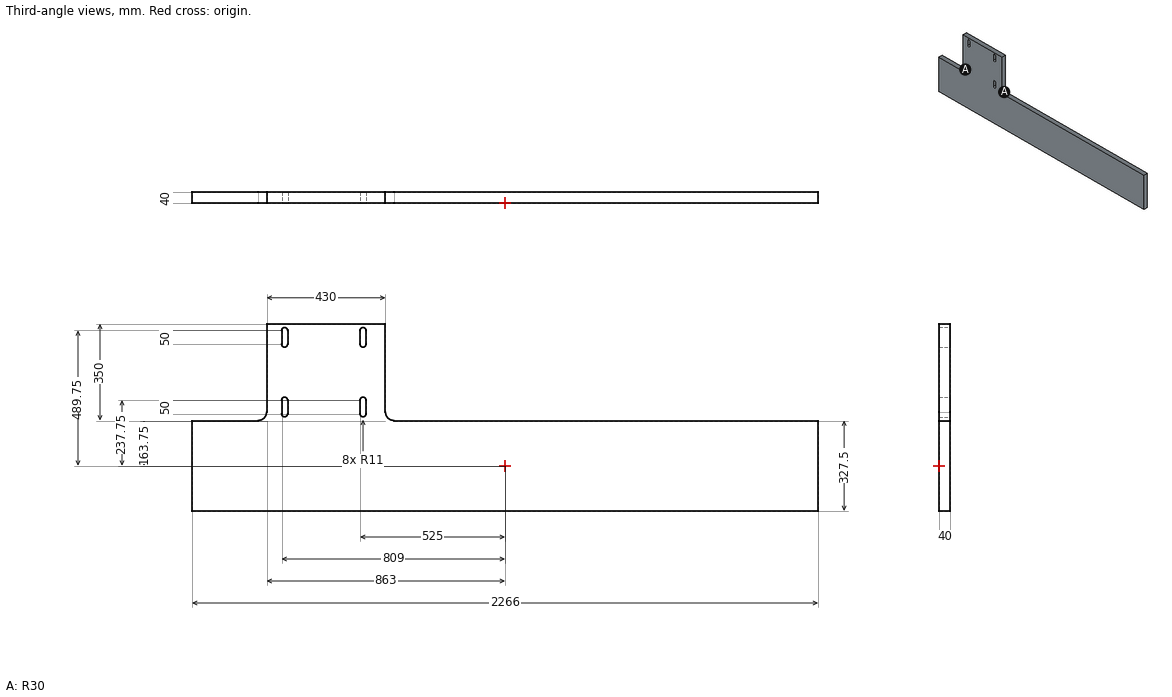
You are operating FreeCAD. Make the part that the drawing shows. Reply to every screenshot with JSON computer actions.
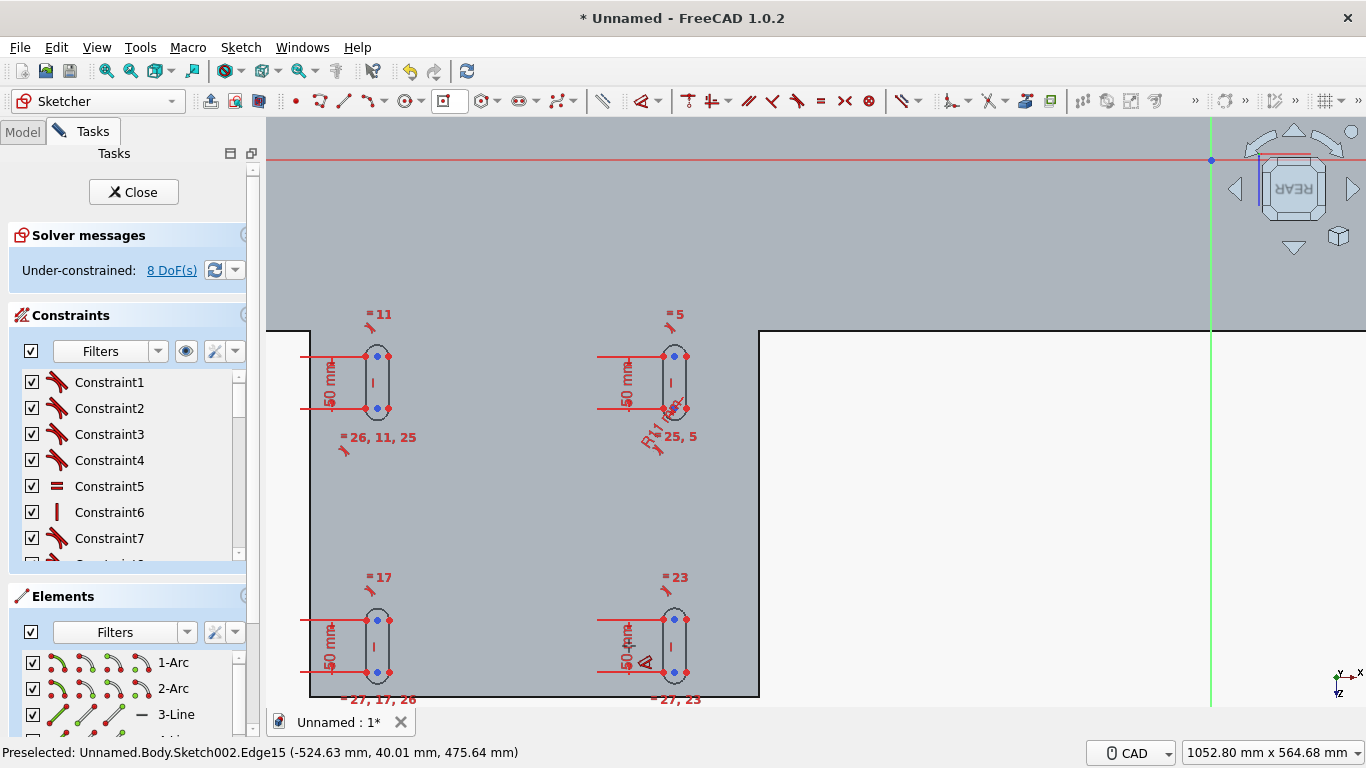
{"action": "left_click", "coordinate": [663, 409]}
{"action": "left_click", "coordinate": [932, 443]}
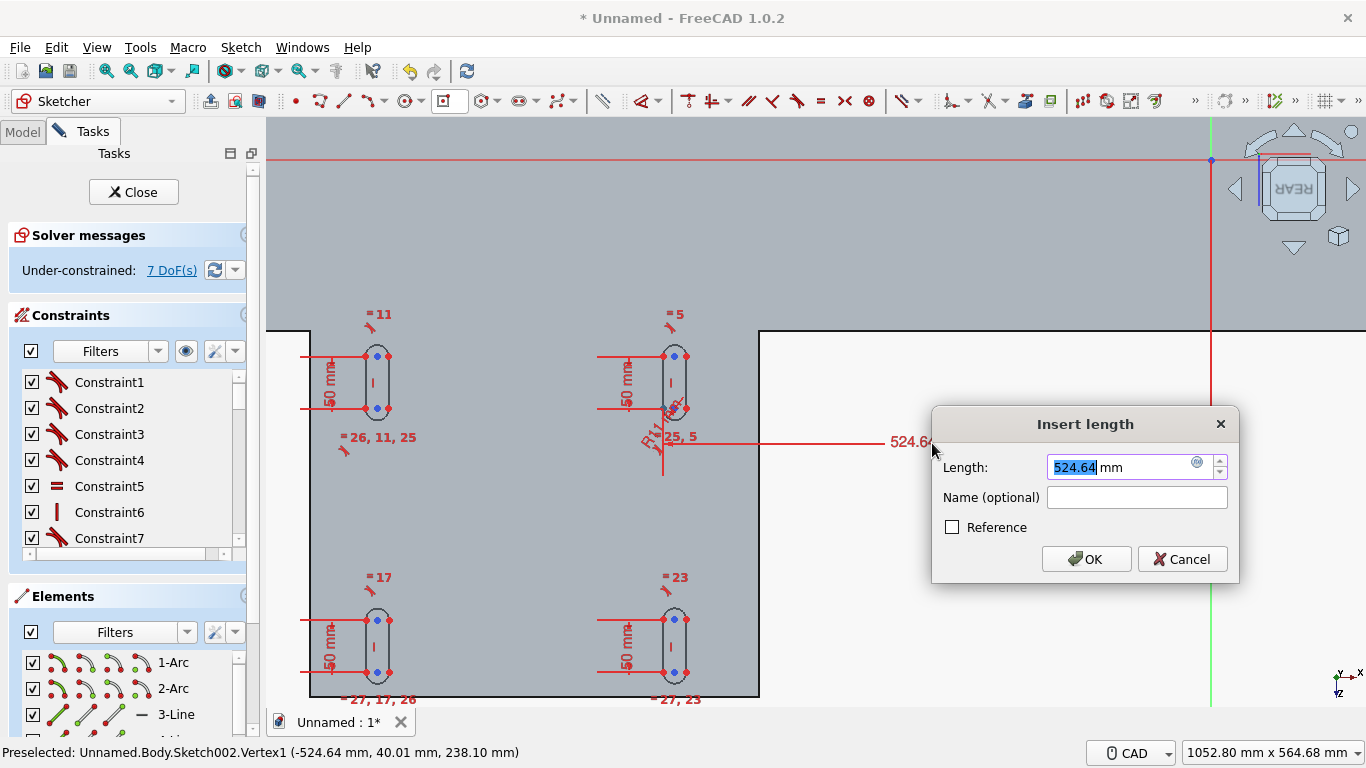
{"action": "type", "text": "525"}
{"action": "key", "text": "Return"}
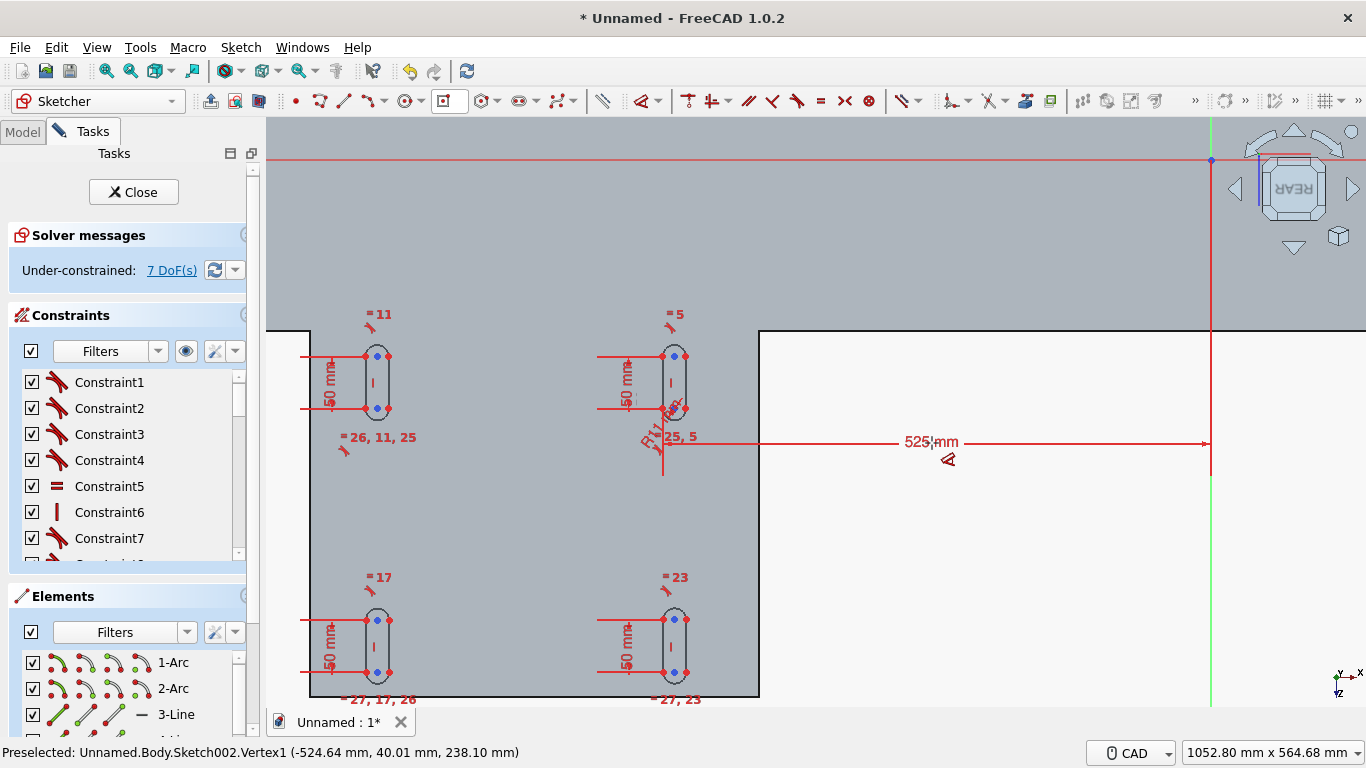
{"action": "left_click", "coordinate": [366, 409]}
{"action": "left_click", "coordinate": [783, 443]}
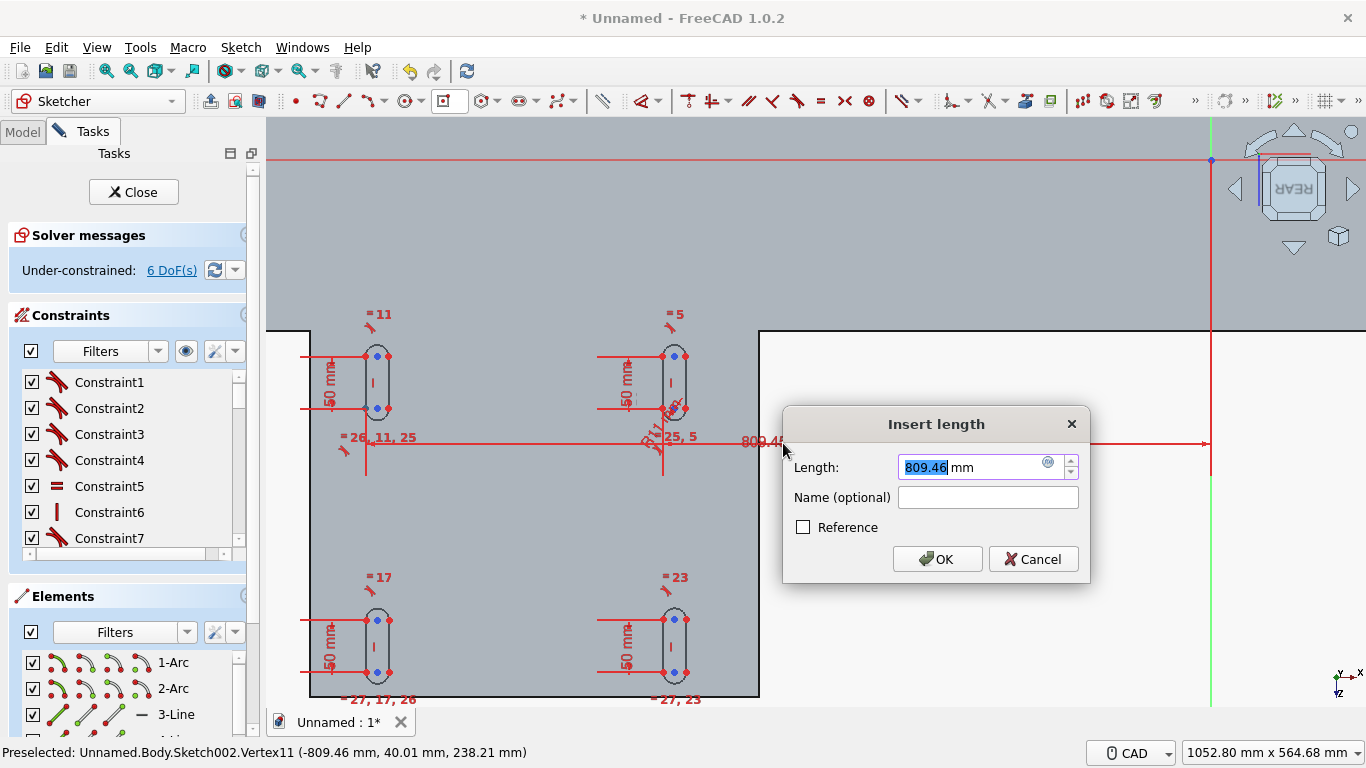
{"action": "type", "text": "809"}
{"action": "key", "text": "Return"}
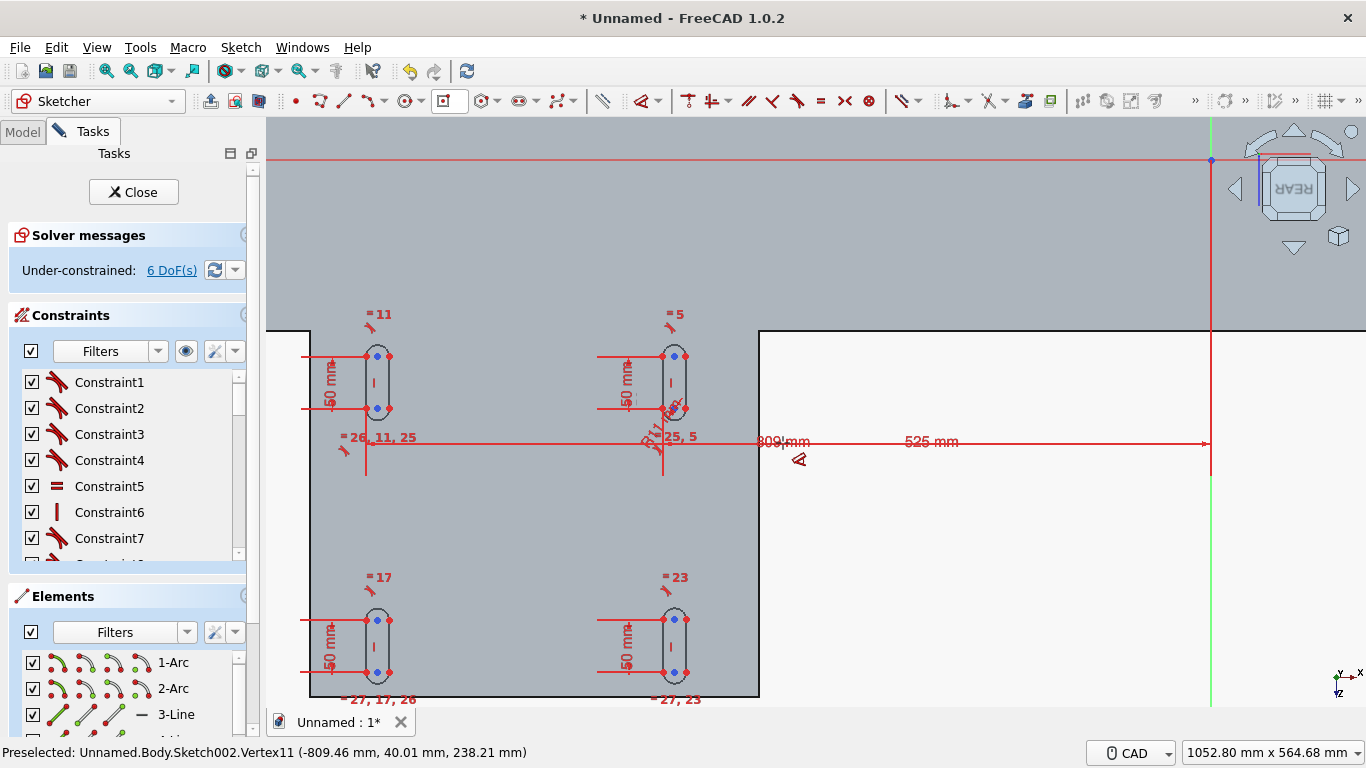
{"action": "left_click", "coordinate": [366, 672]}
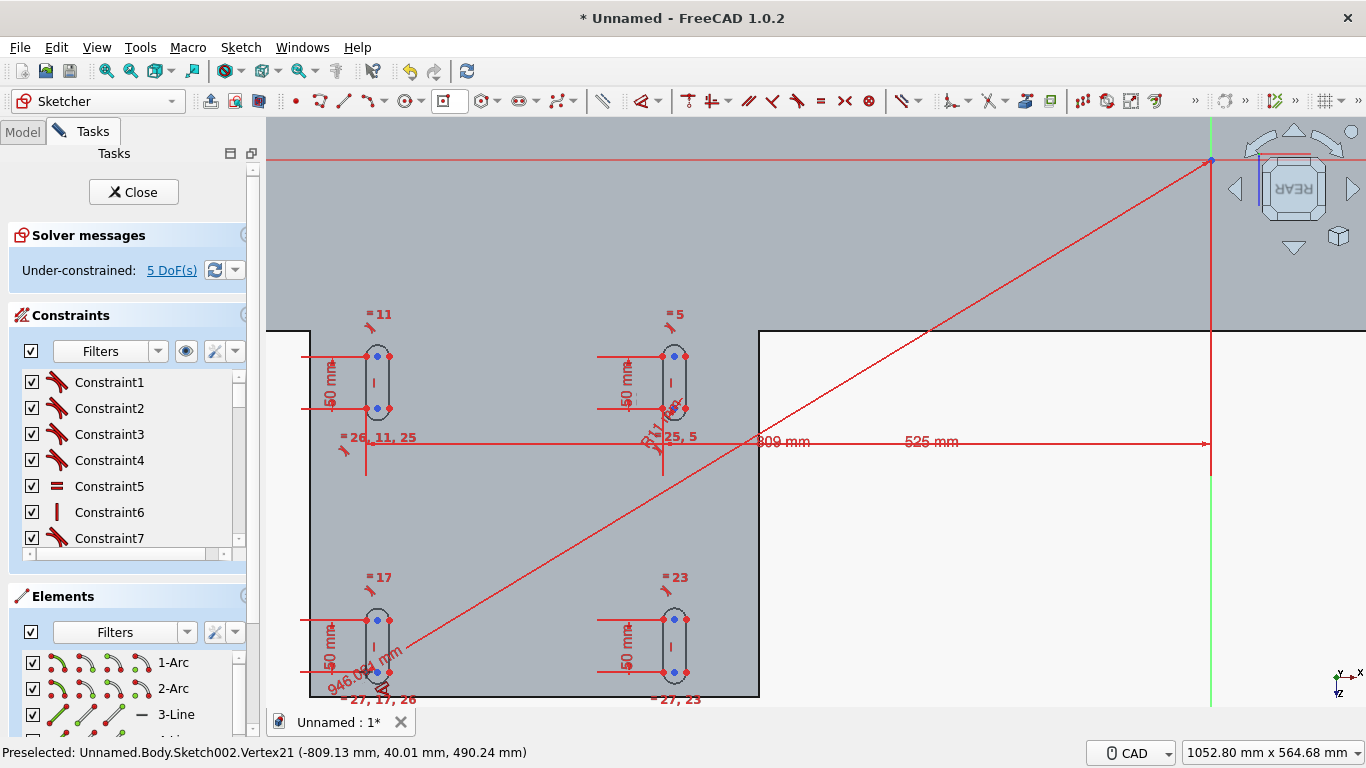
{"action": "key", "text": "Escape"}
{"action": "key", "text": "Escape"}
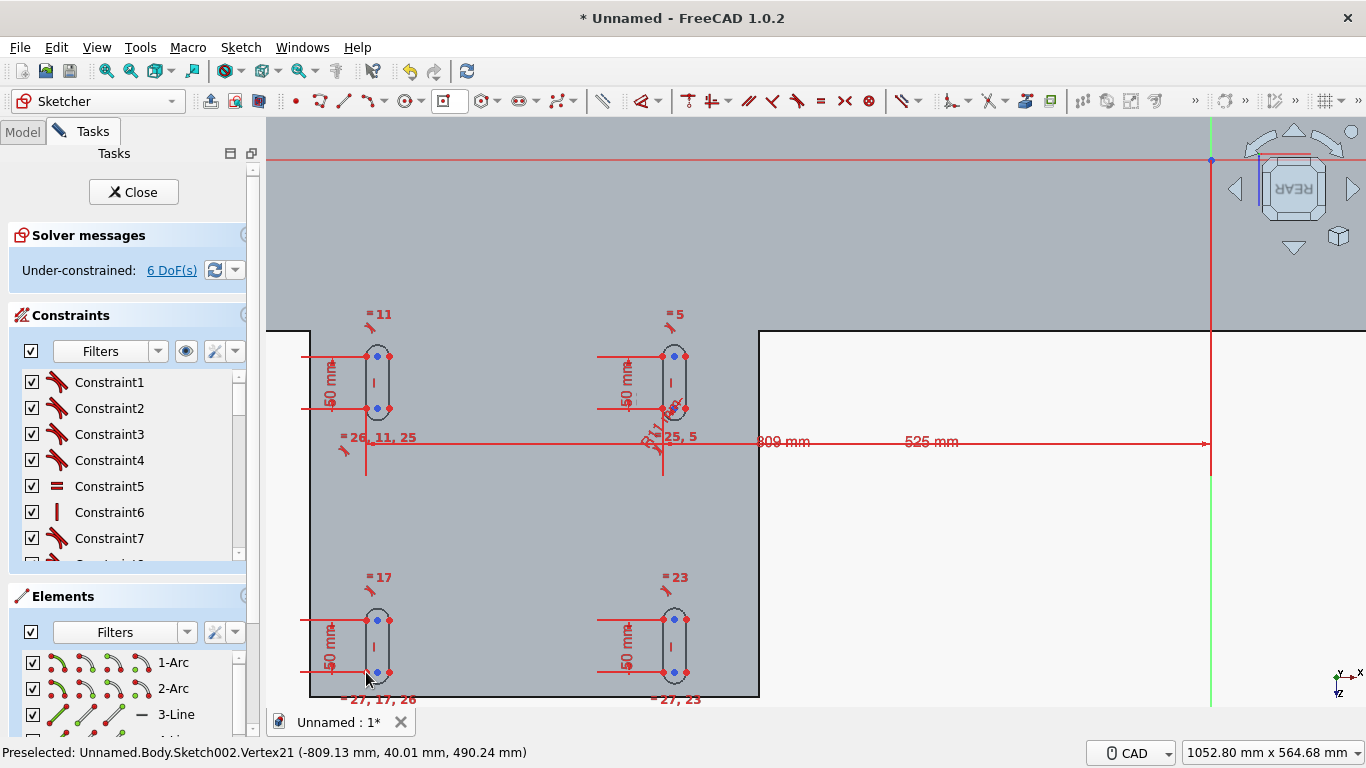
{"action": "left_click", "coordinate": [366, 672]}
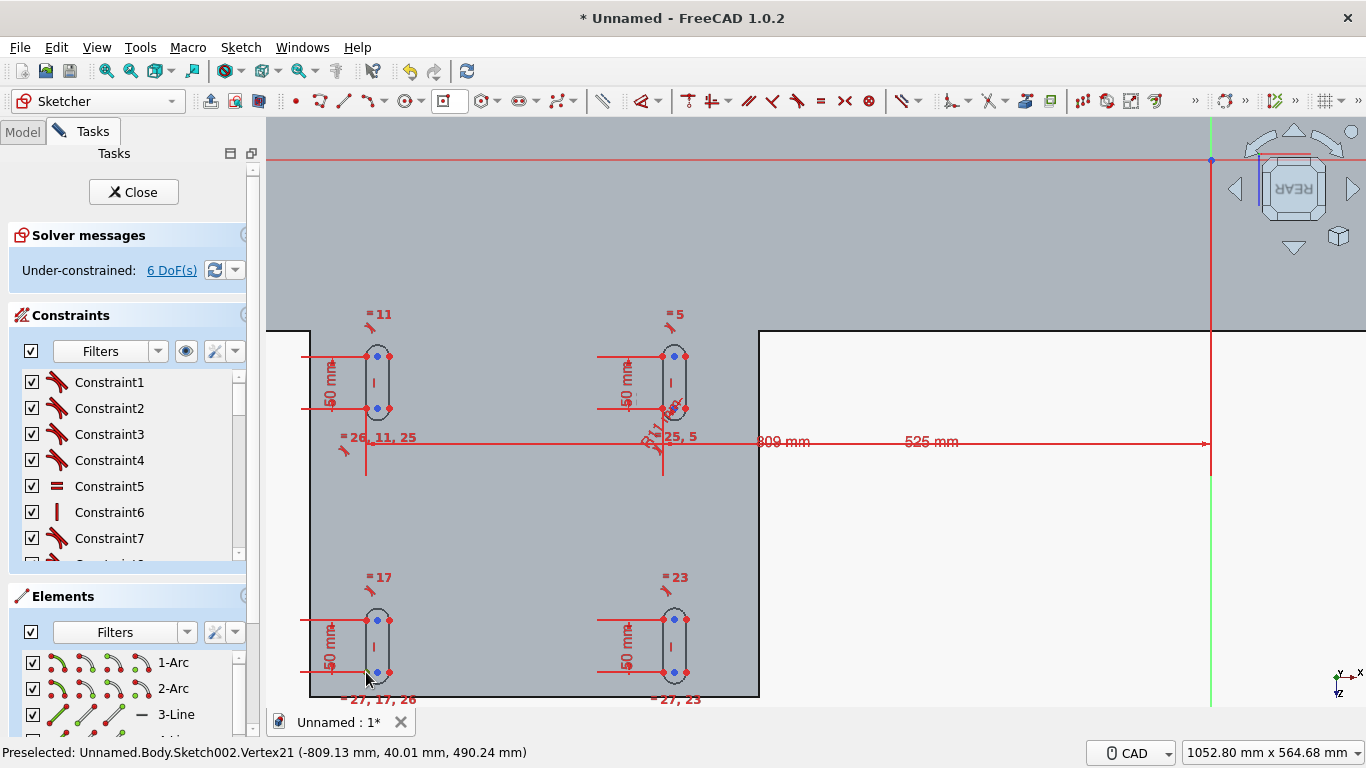
{"action": "left_click", "coordinate": [660, 102]}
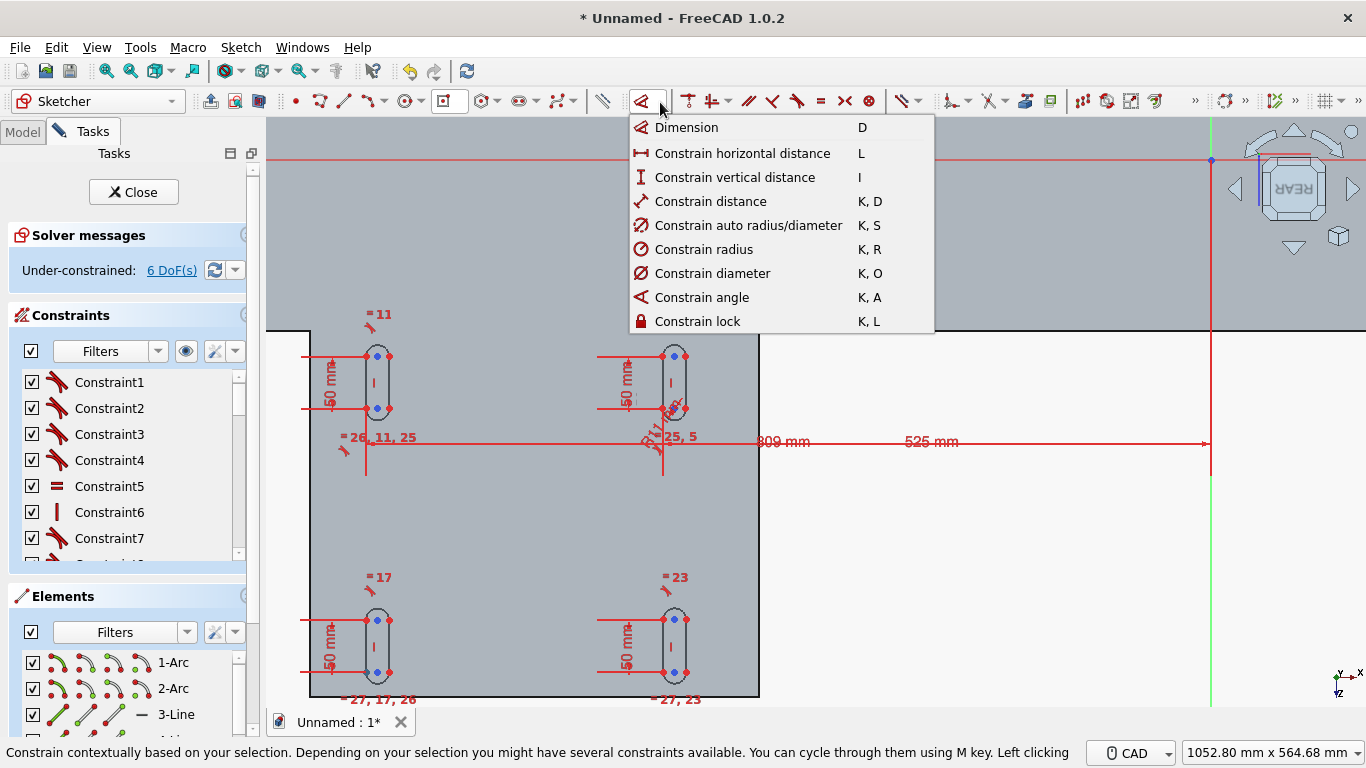
{"action": "left_click", "coordinate": [782, 153]}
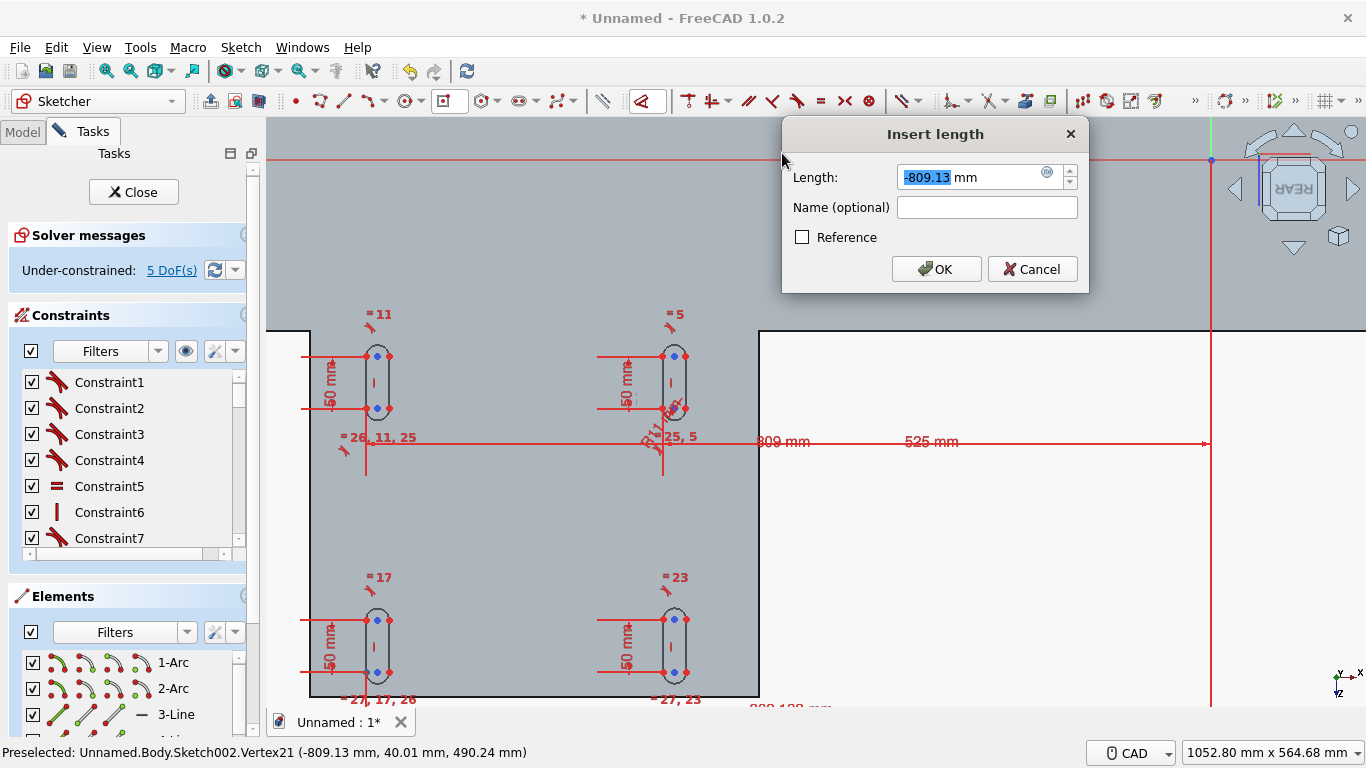
{"action": "type", "text": "-809"}
{"action": "key", "text": "Return"}